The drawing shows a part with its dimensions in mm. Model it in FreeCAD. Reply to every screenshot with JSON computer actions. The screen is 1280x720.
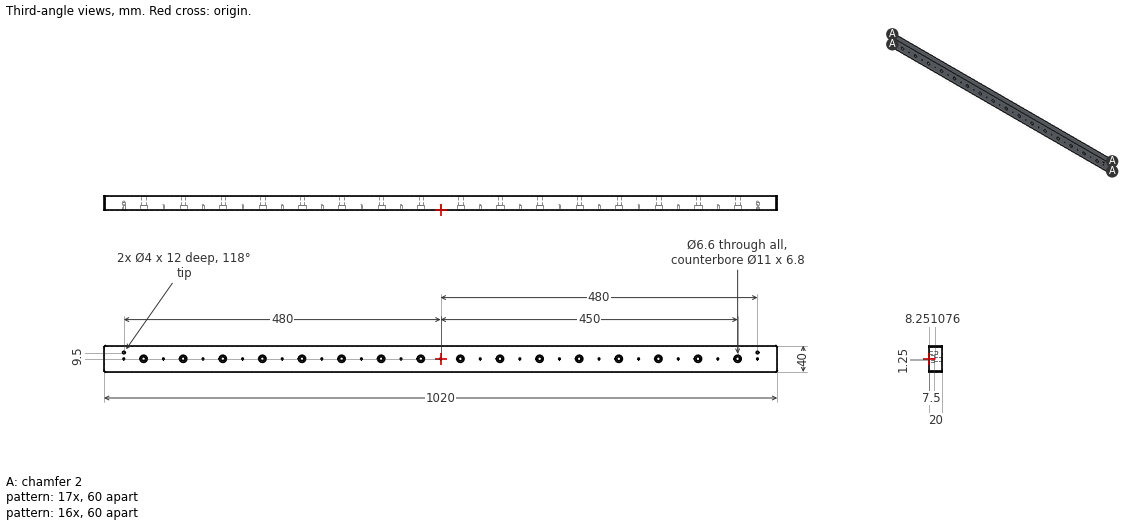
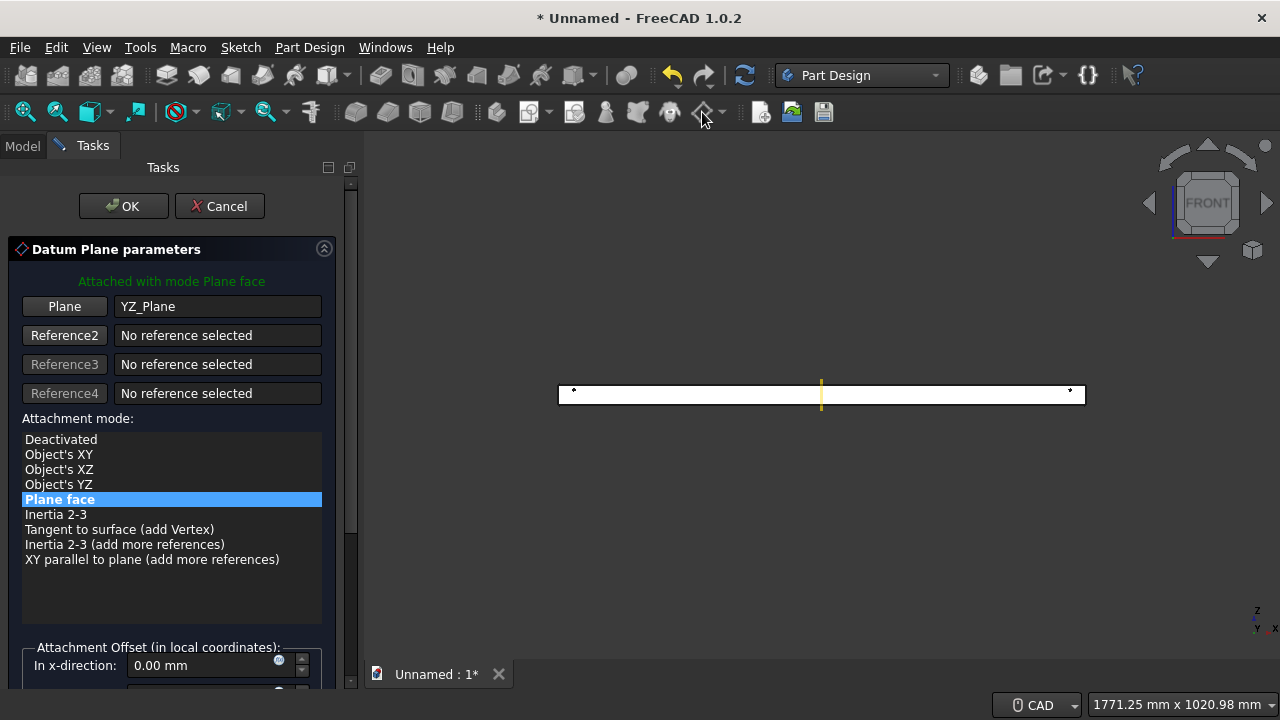
{"action": "scroll", "coordinate": [351, 432], "scroll_direction": "down", "scroll_amount": 2}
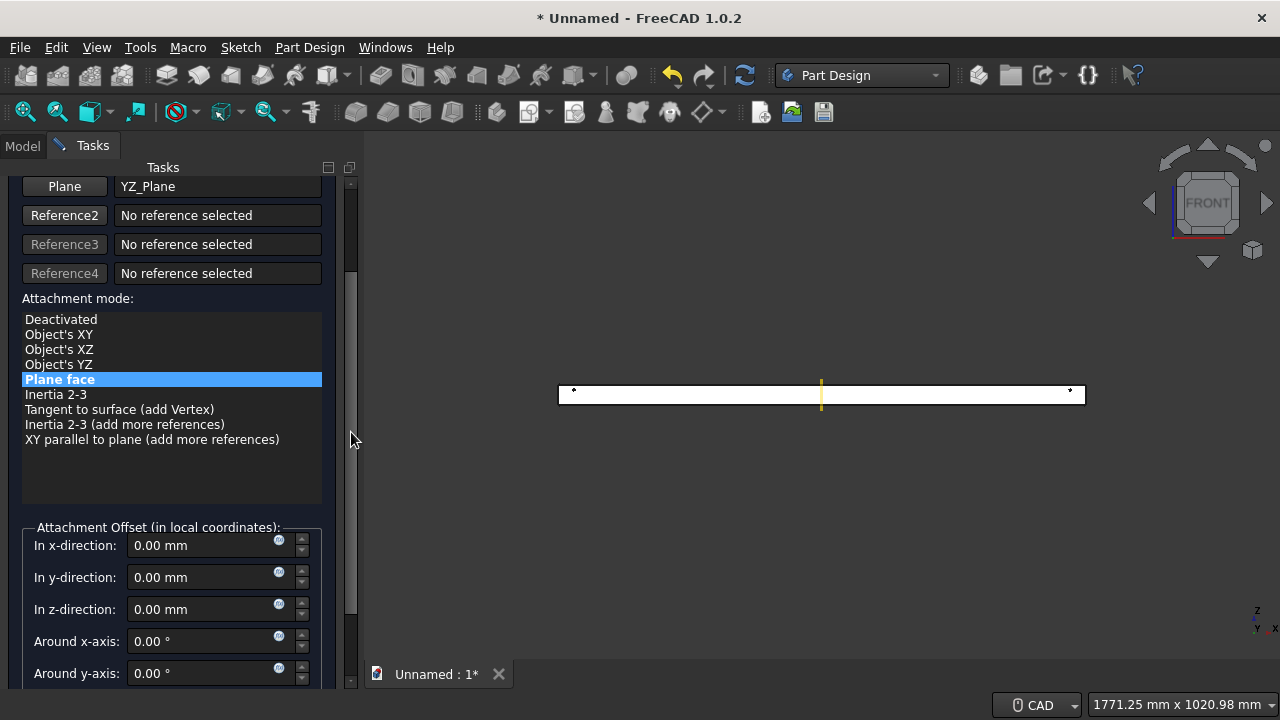
{"action": "triple_click", "coordinate": [210, 609]}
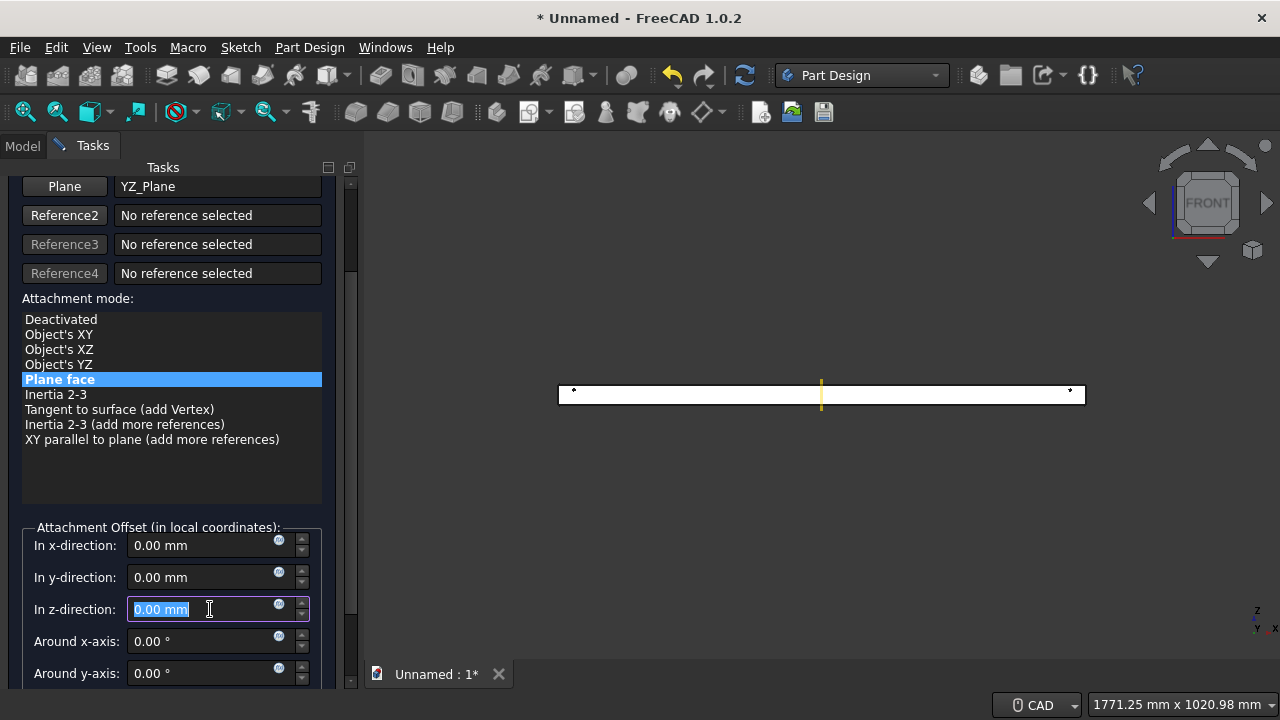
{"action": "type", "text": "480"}
{"action": "key", "text": "Tab"}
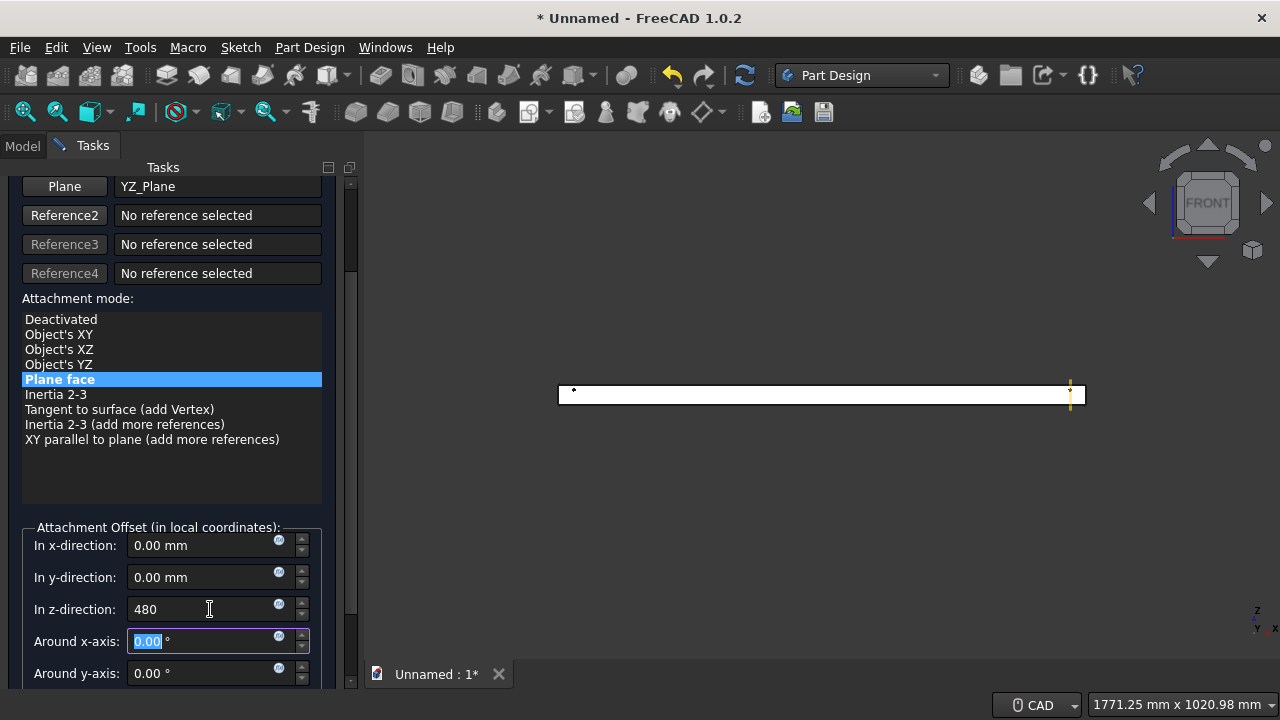
{"action": "scroll", "coordinate": [351, 432], "scroll_direction": "up", "scroll_amount": 3}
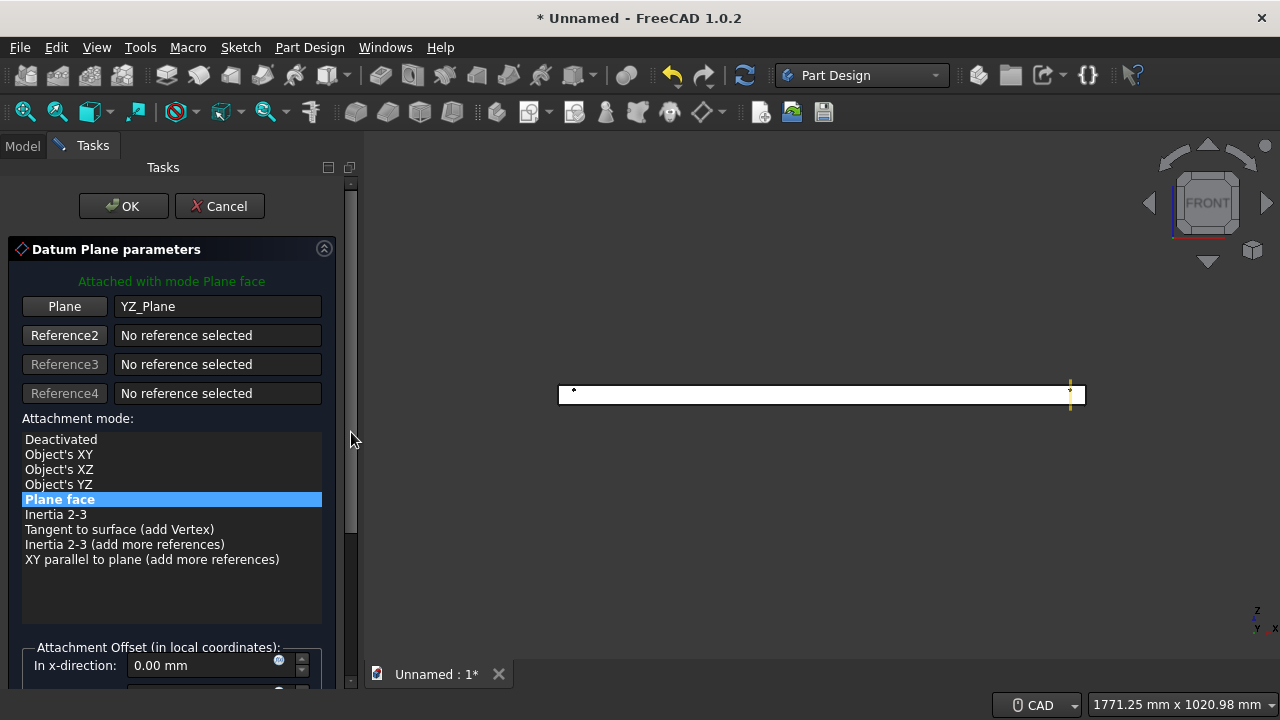
{"action": "left_click", "coordinate": [124, 206]}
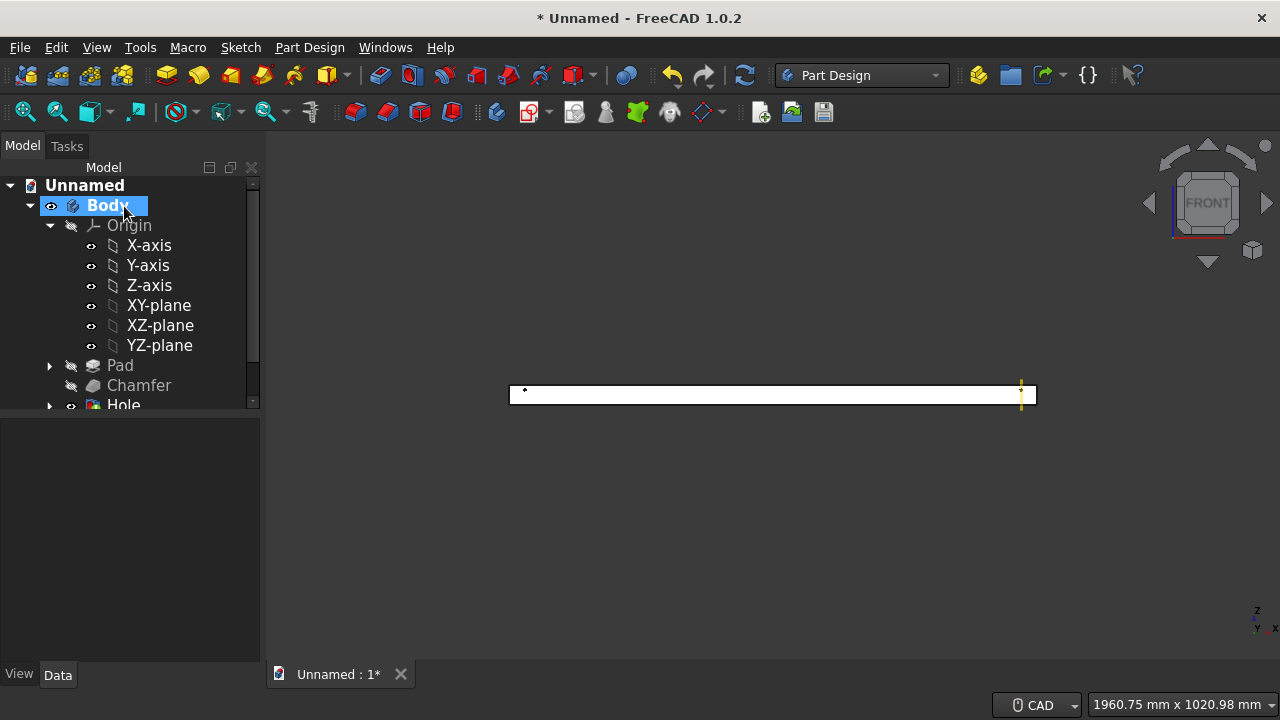
{"action": "scroll", "coordinate": [100, 301], "scroll_direction": "down", "scroll_amount": 3}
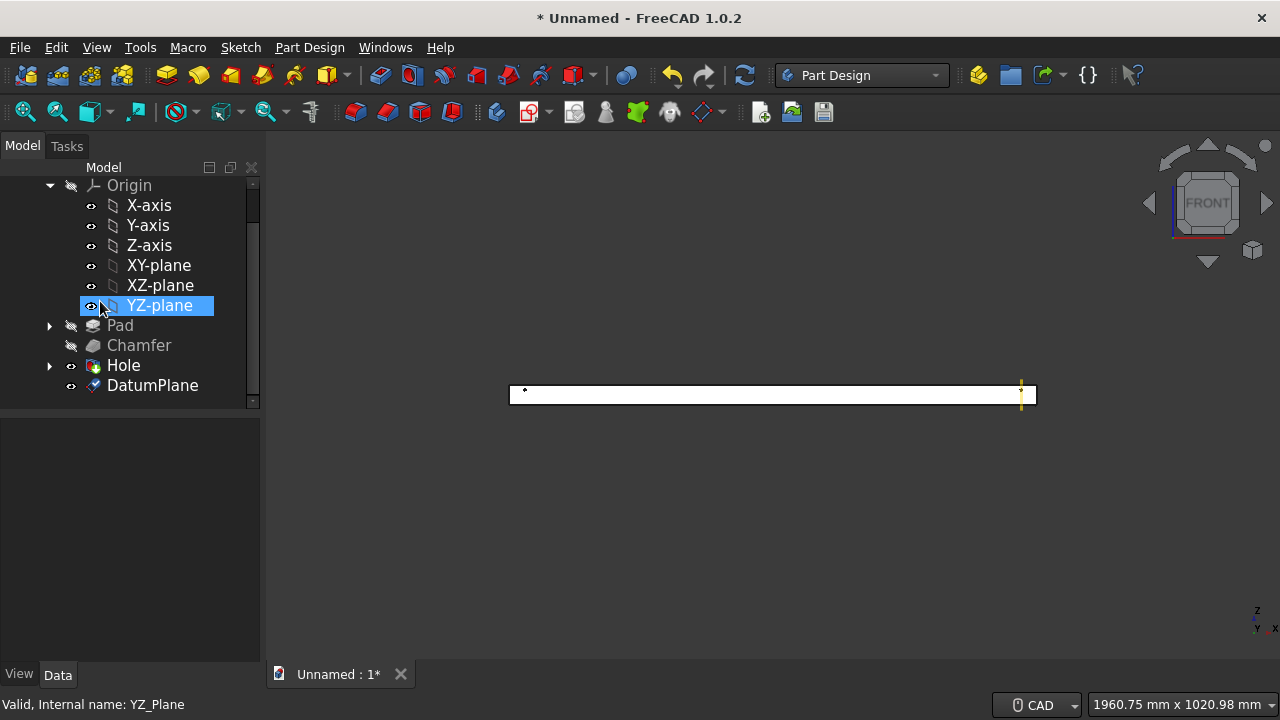
{"action": "left_click", "coordinate": [116, 386]}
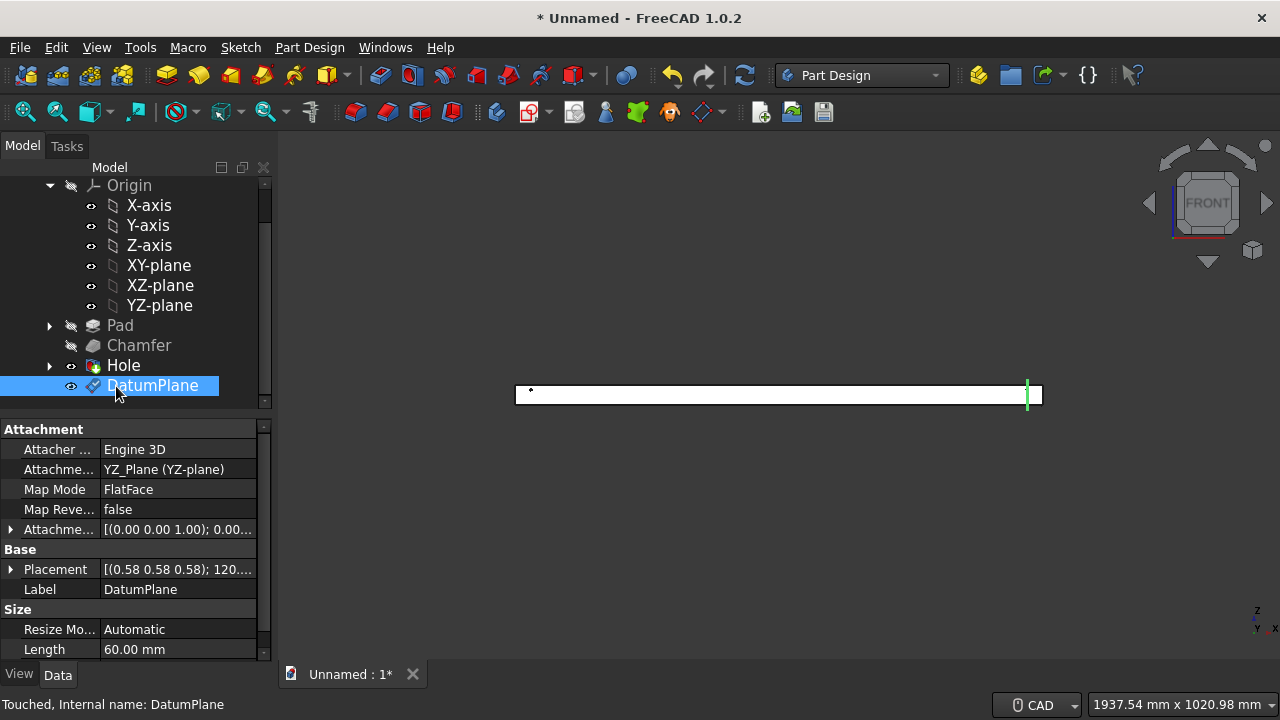
{"action": "left_click", "coordinate": [530, 112]}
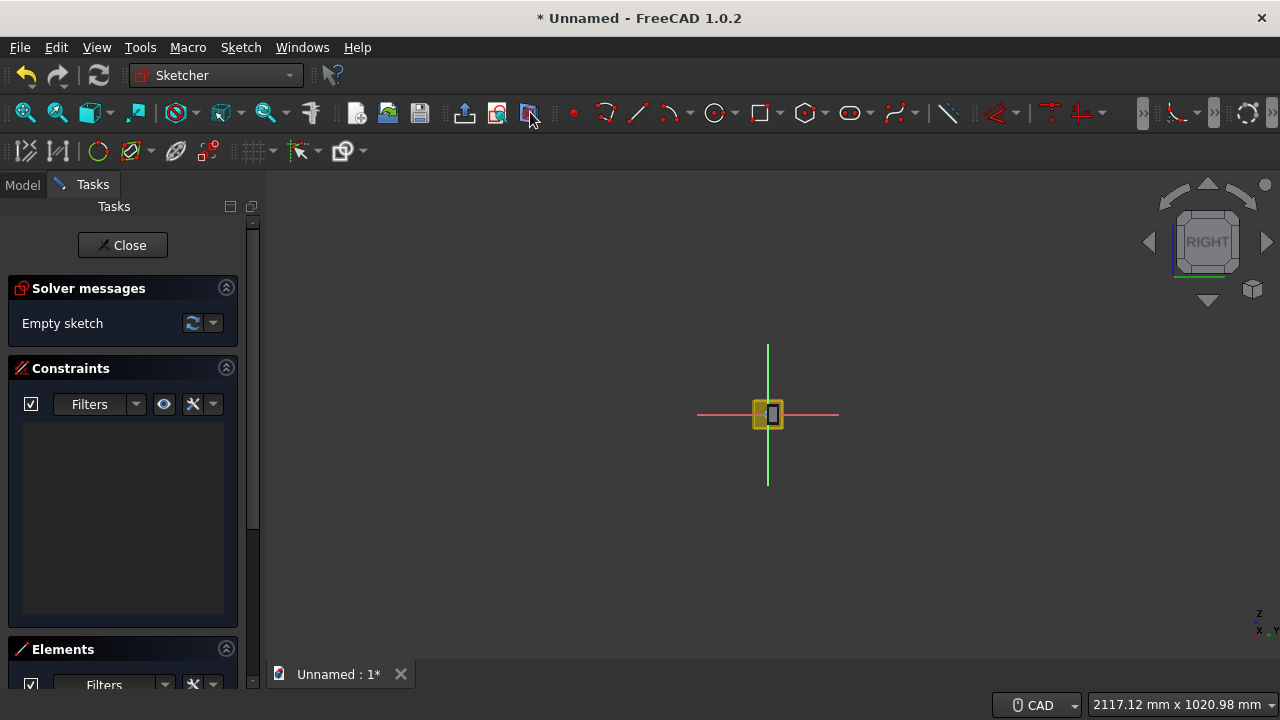
{"action": "key", "text": "q s"}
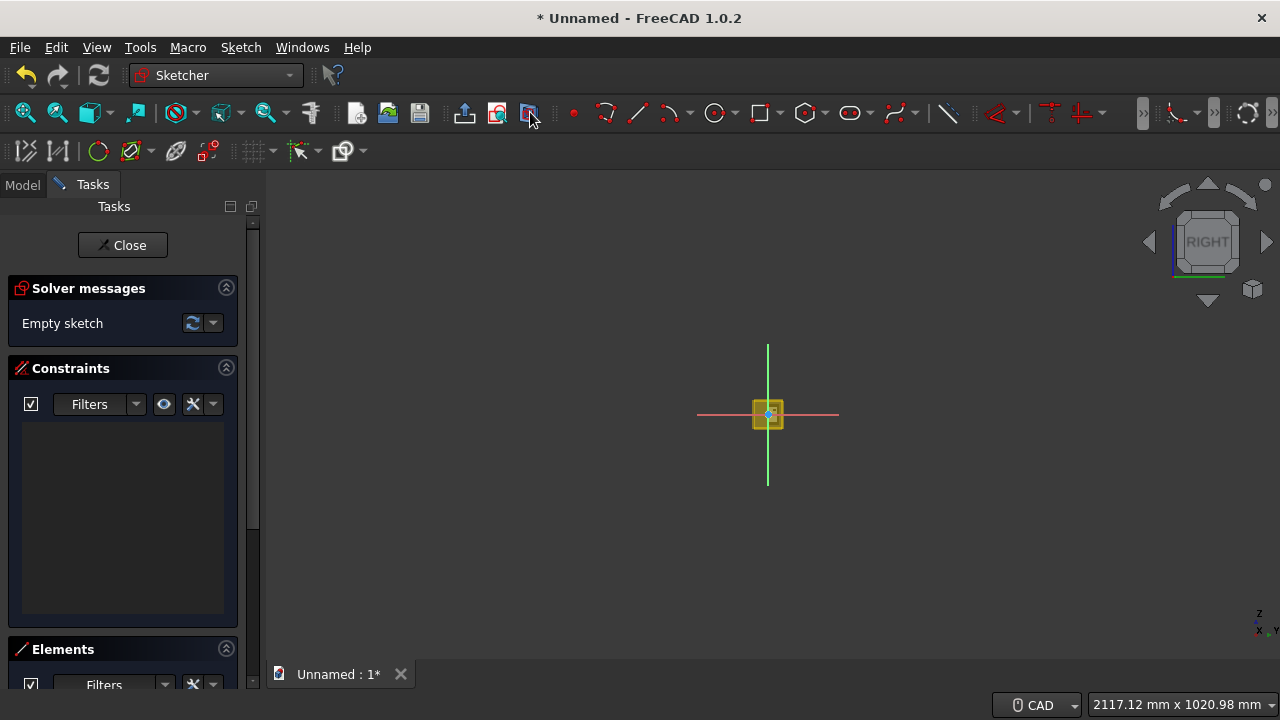
{"action": "scroll", "coordinate": [774, 415], "scroll_direction": "up", "scroll_amount": 15}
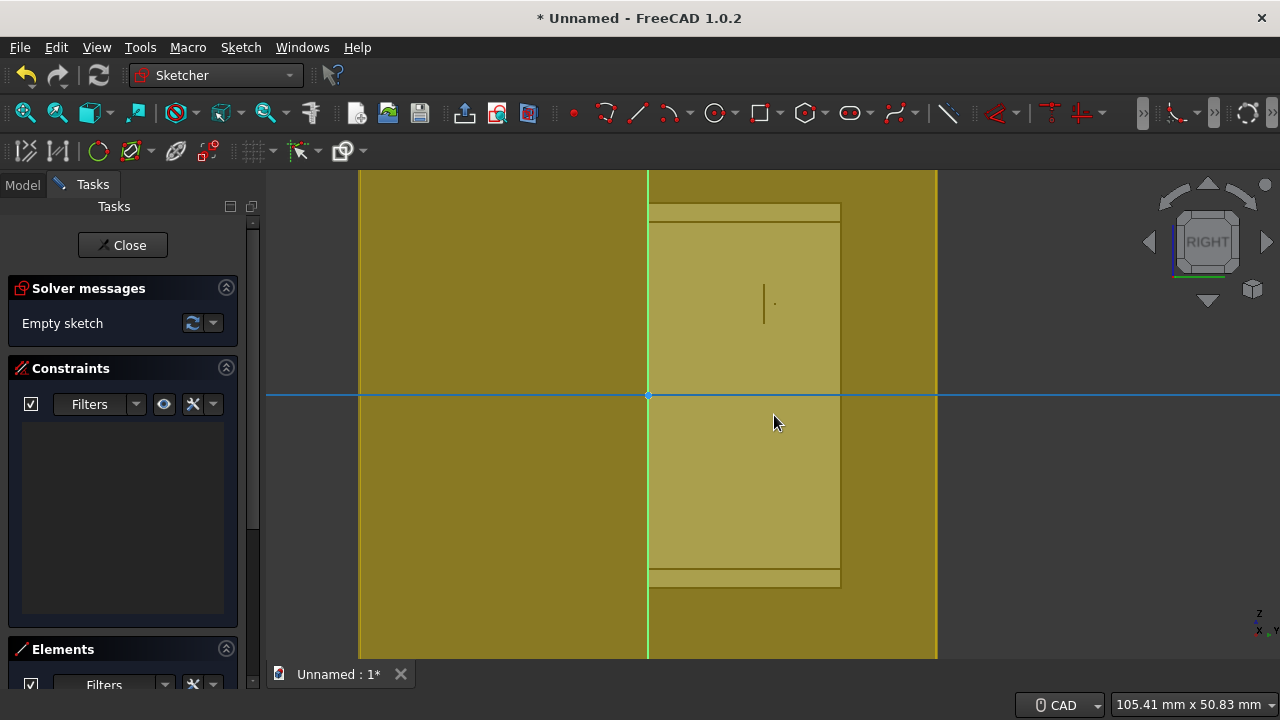
{"action": "scroll", "coordinate": [685, 399], "scroll_direction": "up", "scroll_amount": 10}